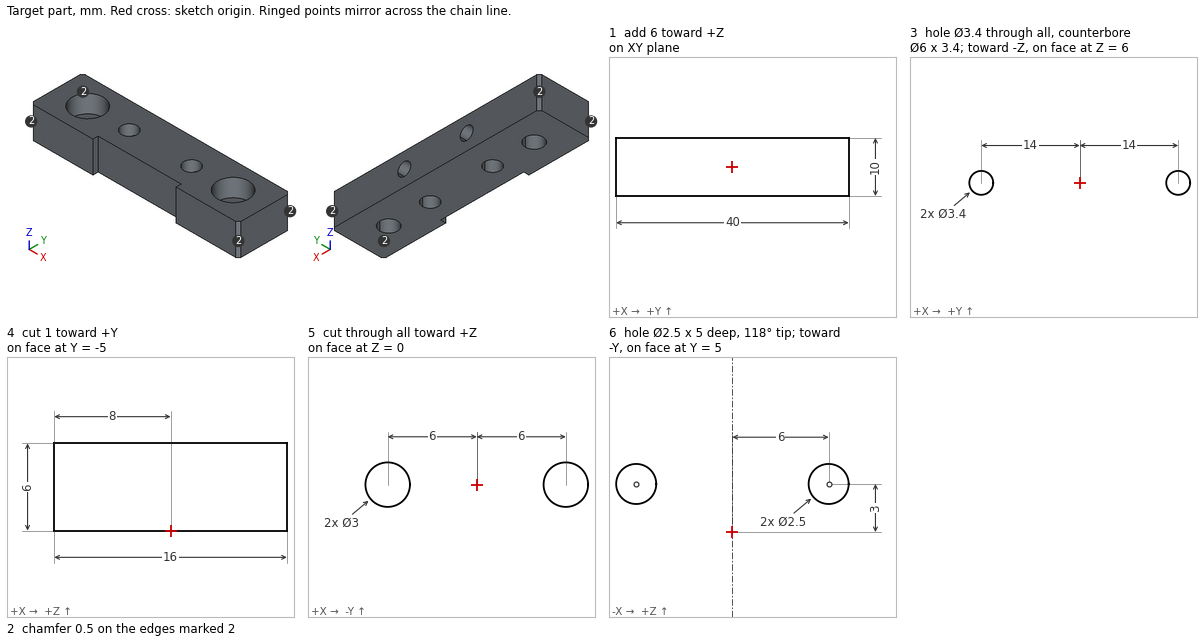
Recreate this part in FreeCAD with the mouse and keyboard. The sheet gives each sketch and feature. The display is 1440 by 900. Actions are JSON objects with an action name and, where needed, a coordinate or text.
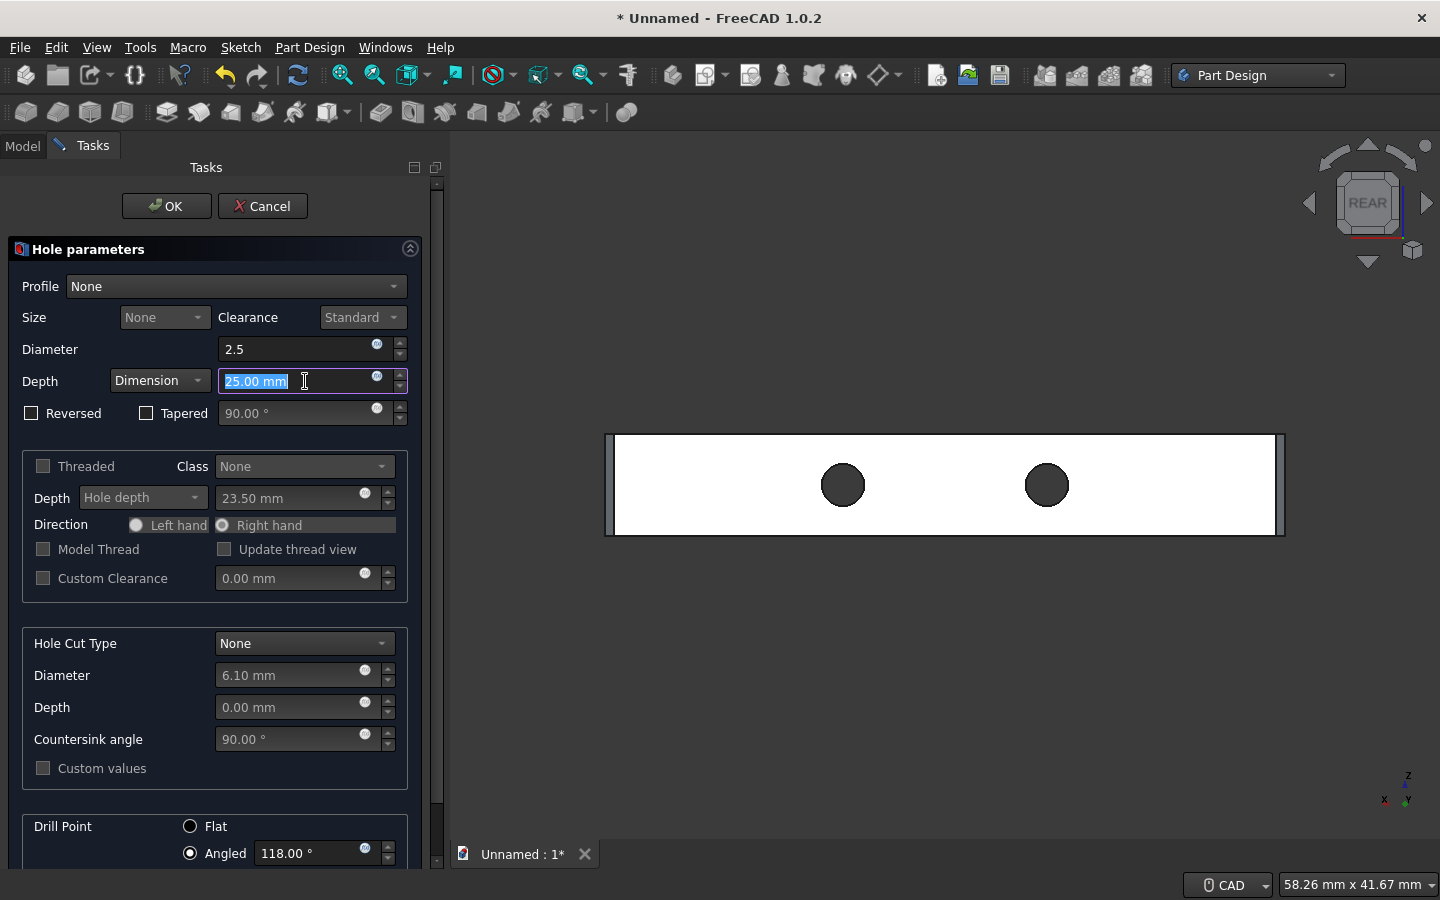
{"action": "type", "text": "5"}
{"action": "key", "text": "Tab"}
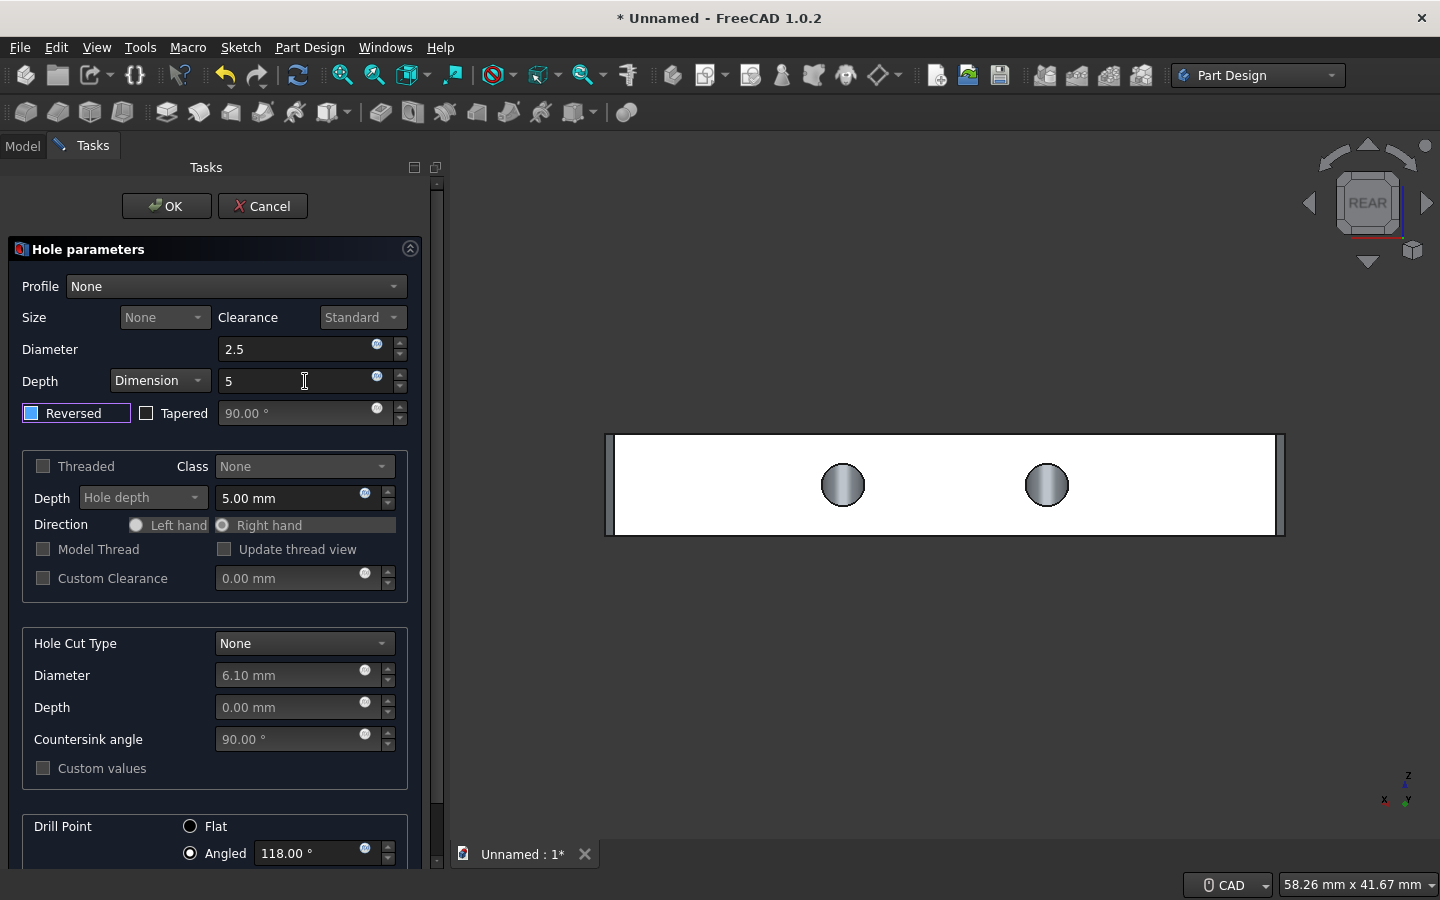
{"action": "left_click", "coordinate": [167, 206]}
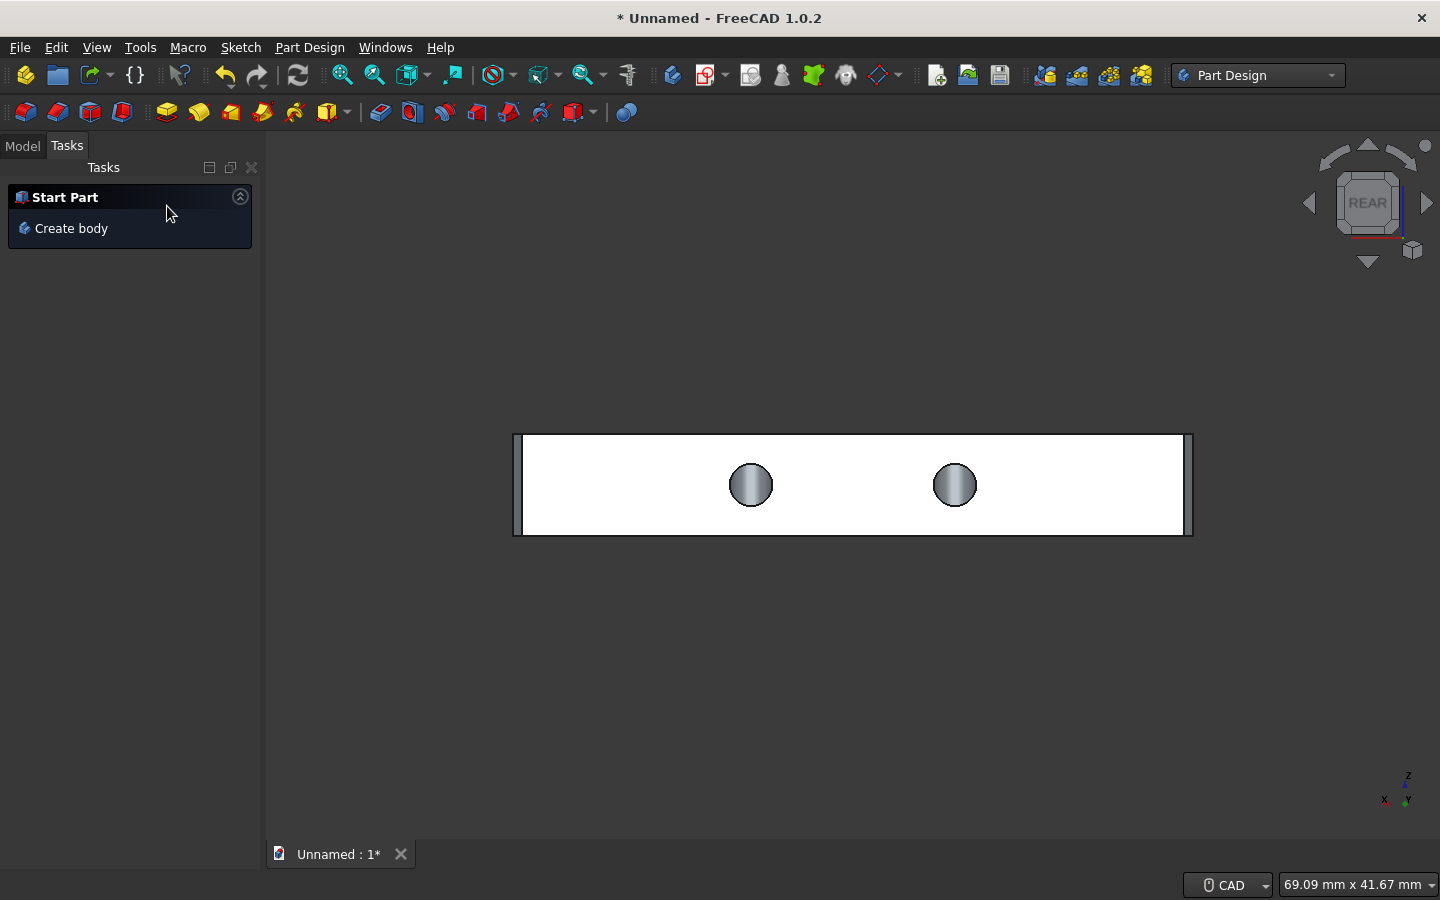
{"action": "key", "text": "0"}